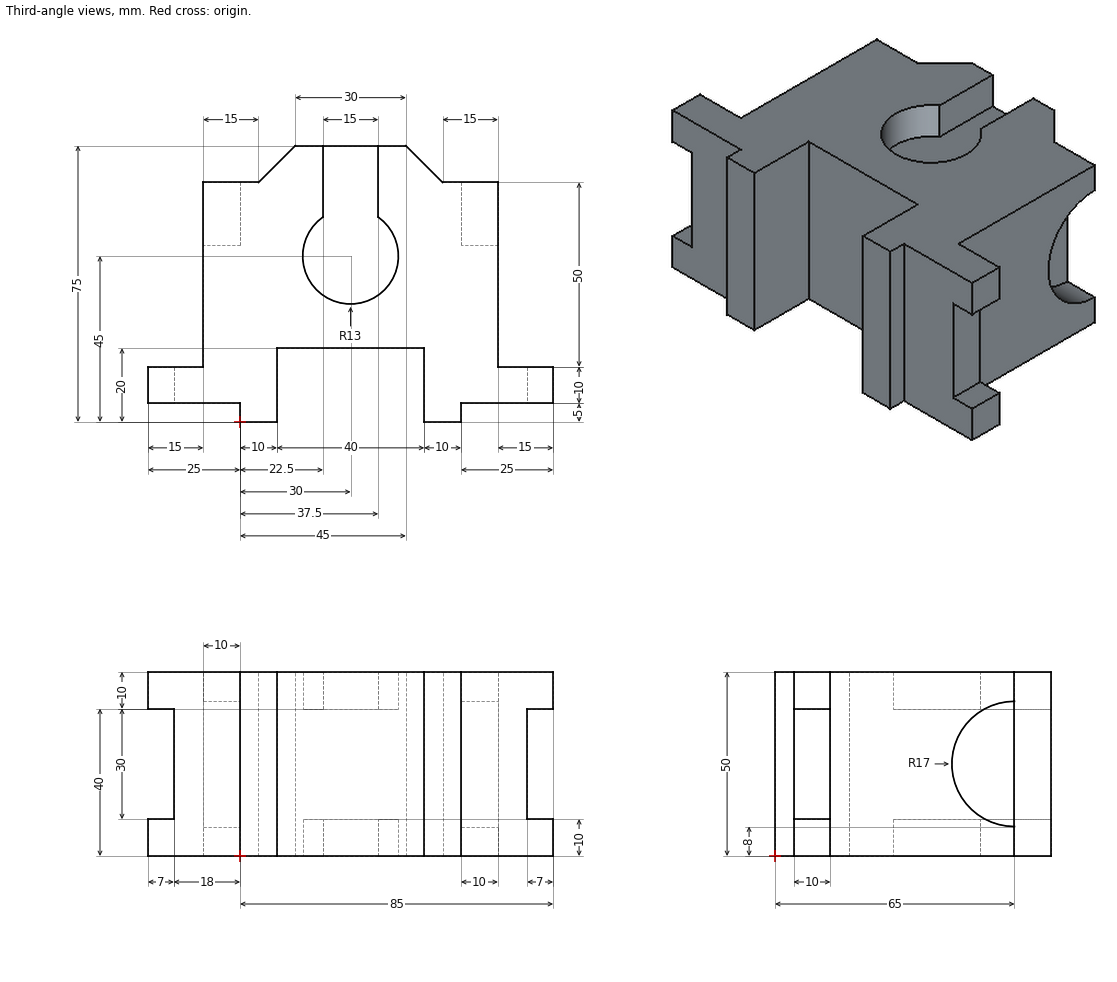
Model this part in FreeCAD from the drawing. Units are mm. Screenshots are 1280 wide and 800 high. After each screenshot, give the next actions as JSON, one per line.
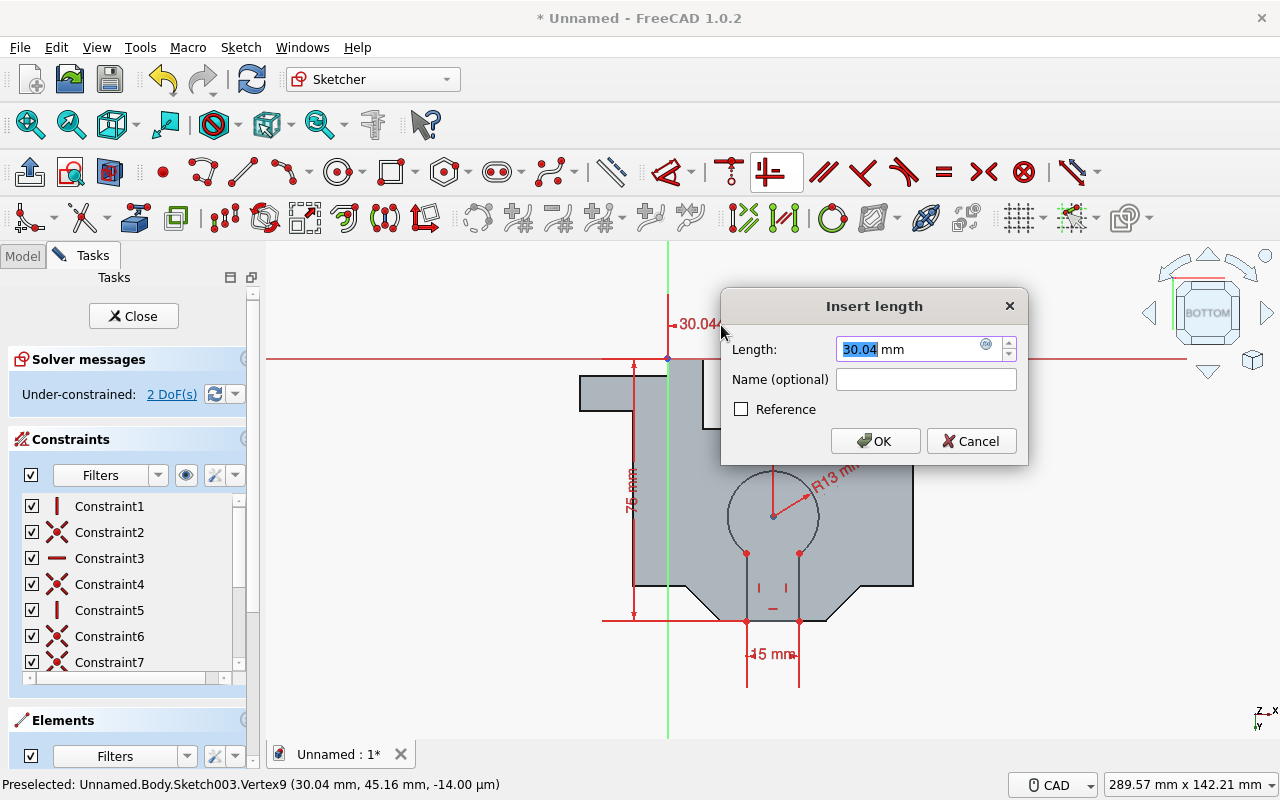
{"action": "type", "text": "30"}
{"action": "key", "text": "Return"}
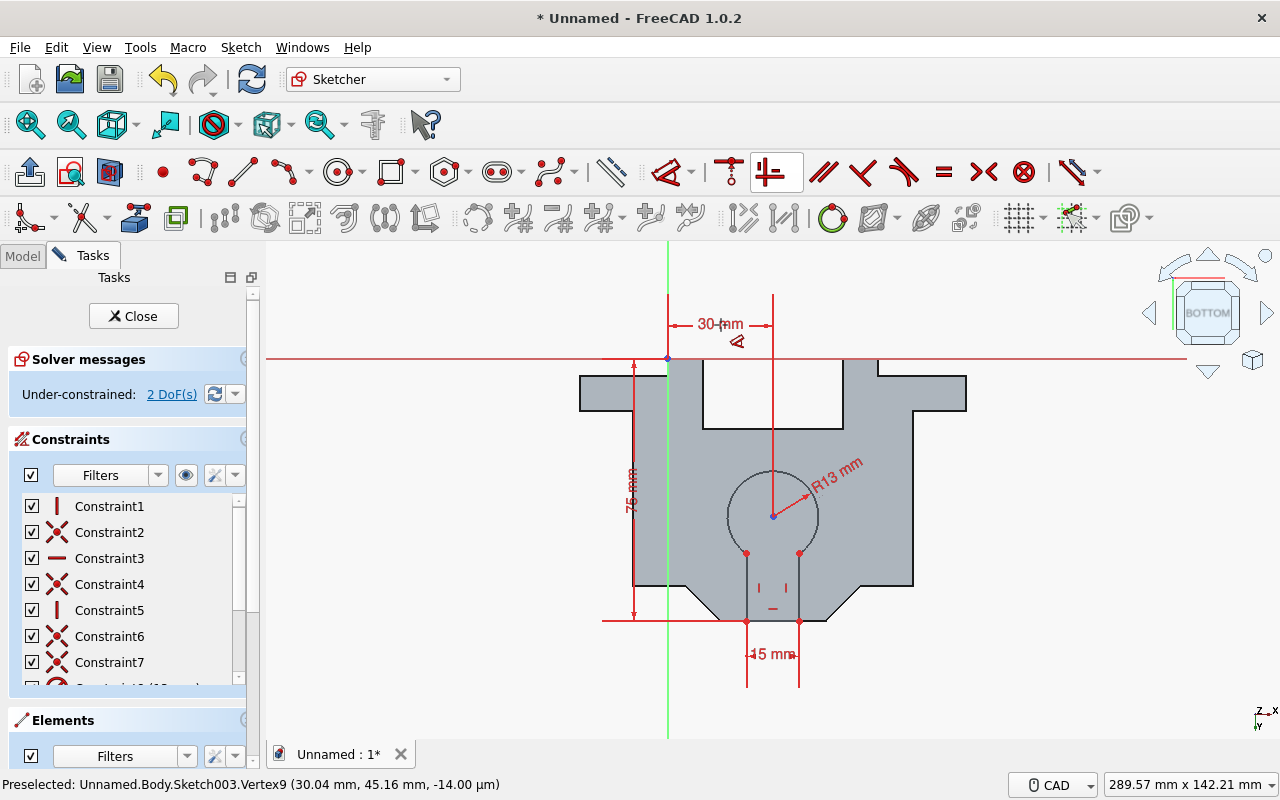
{"action": "left_click", "coordinate": [773, 517]}
{"action": "left_click", "coordinate": [634, 438]}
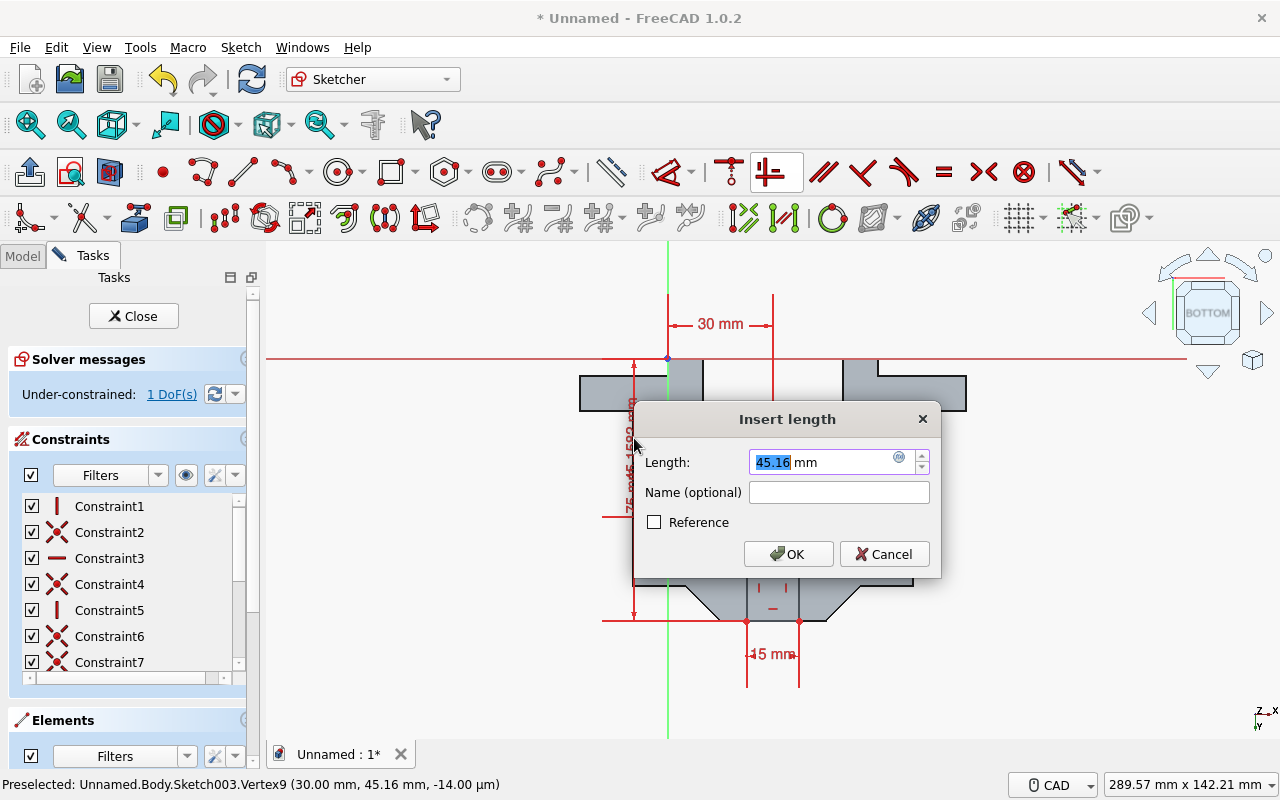
{"action": "type", "text": "45"}
{"action": "key", "text": "Return"}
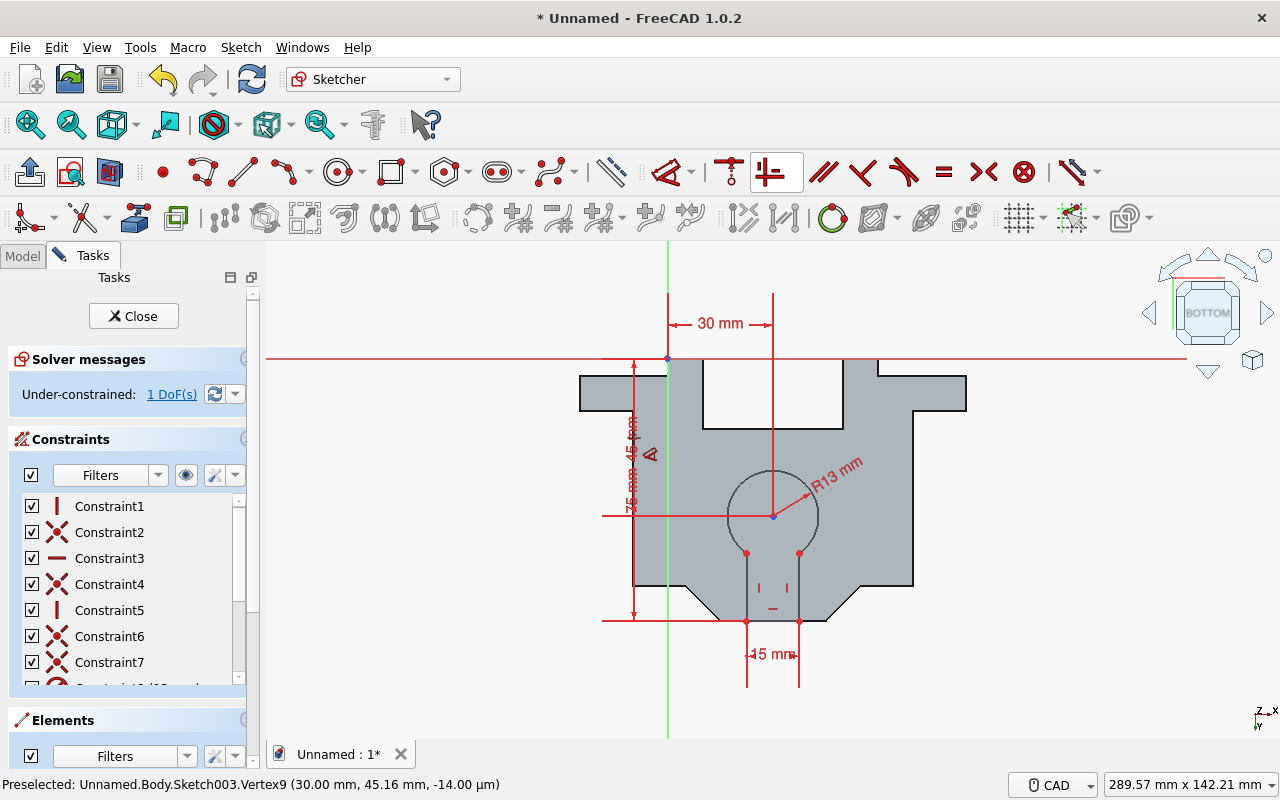
{"action": "left_click", "coordinate": [747, 554]}
{"action": "left_click", "coordinate": [707, 588]}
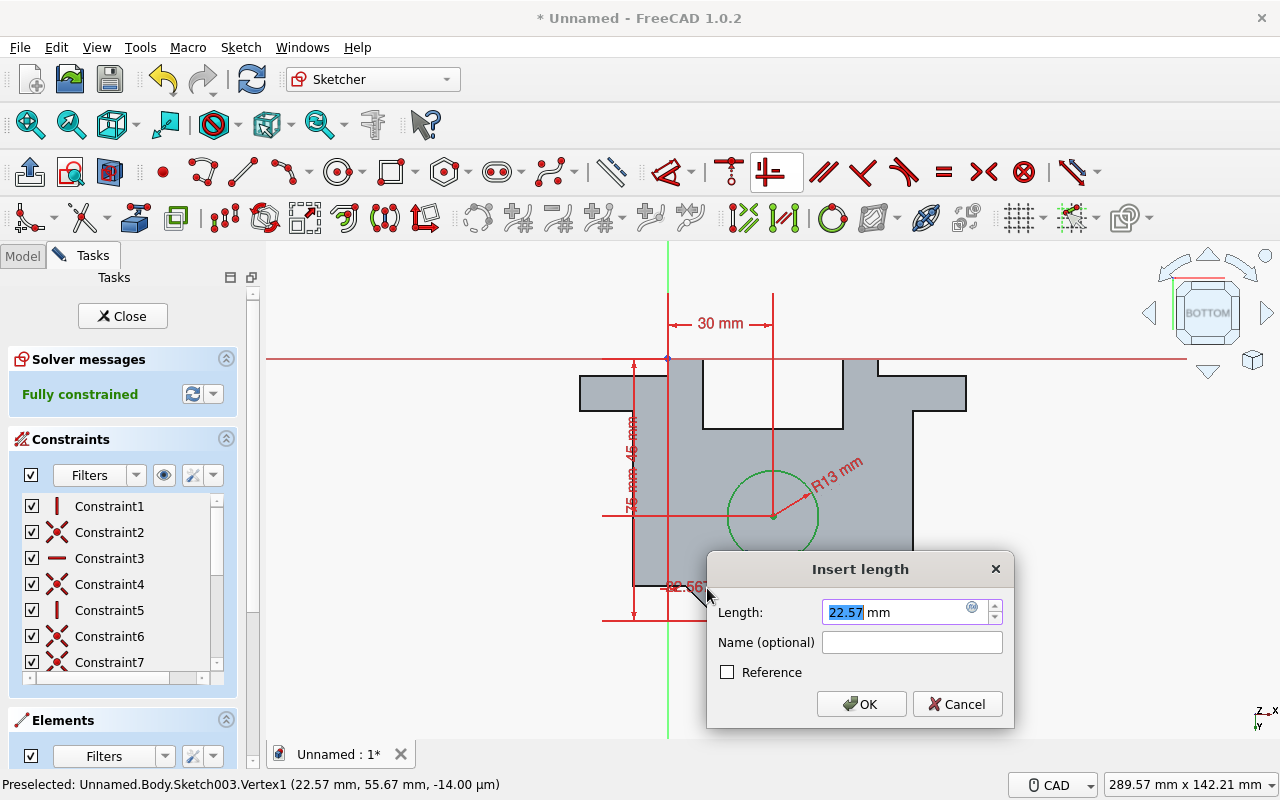
{"action": "type", "text": "22.5"}
{"action": "key", "text": "Return"}
{"action": "key", "text": "Escape"}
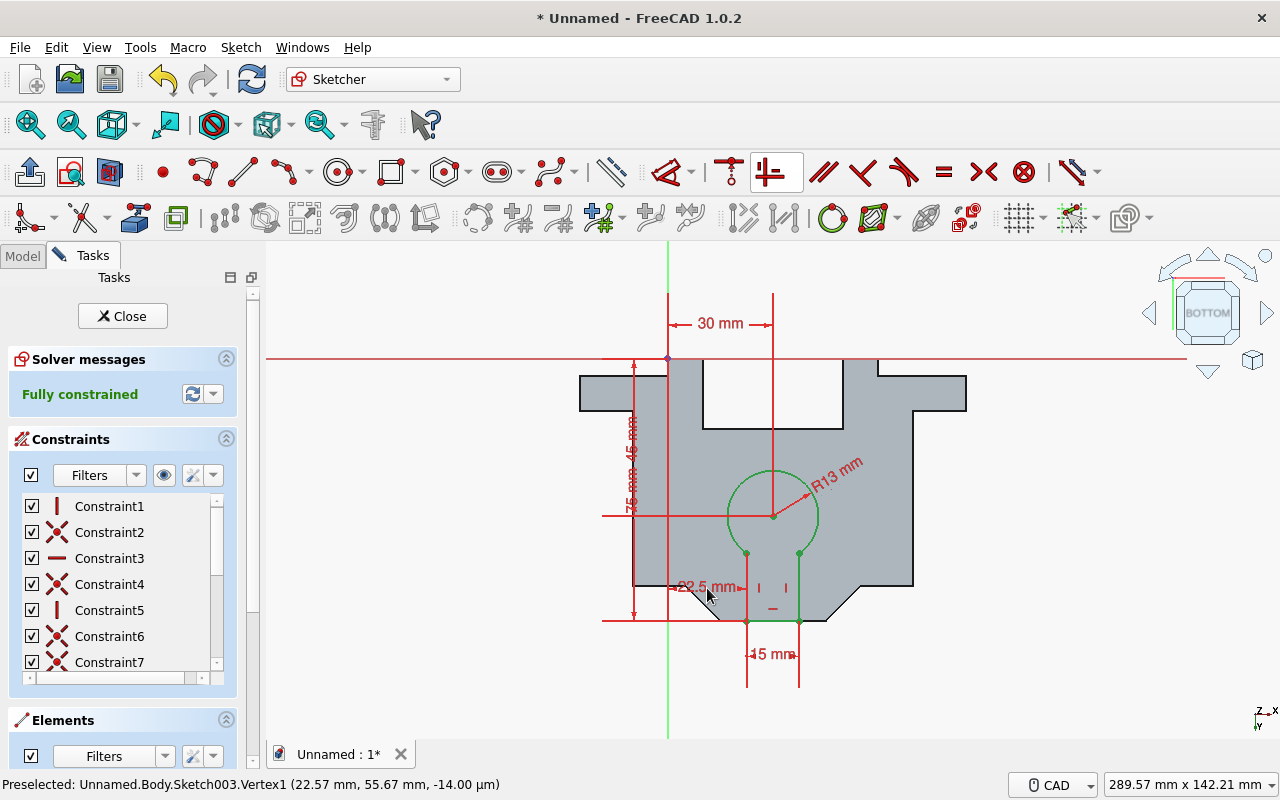
{"action": "left_click", "coordinate": [123, 316]}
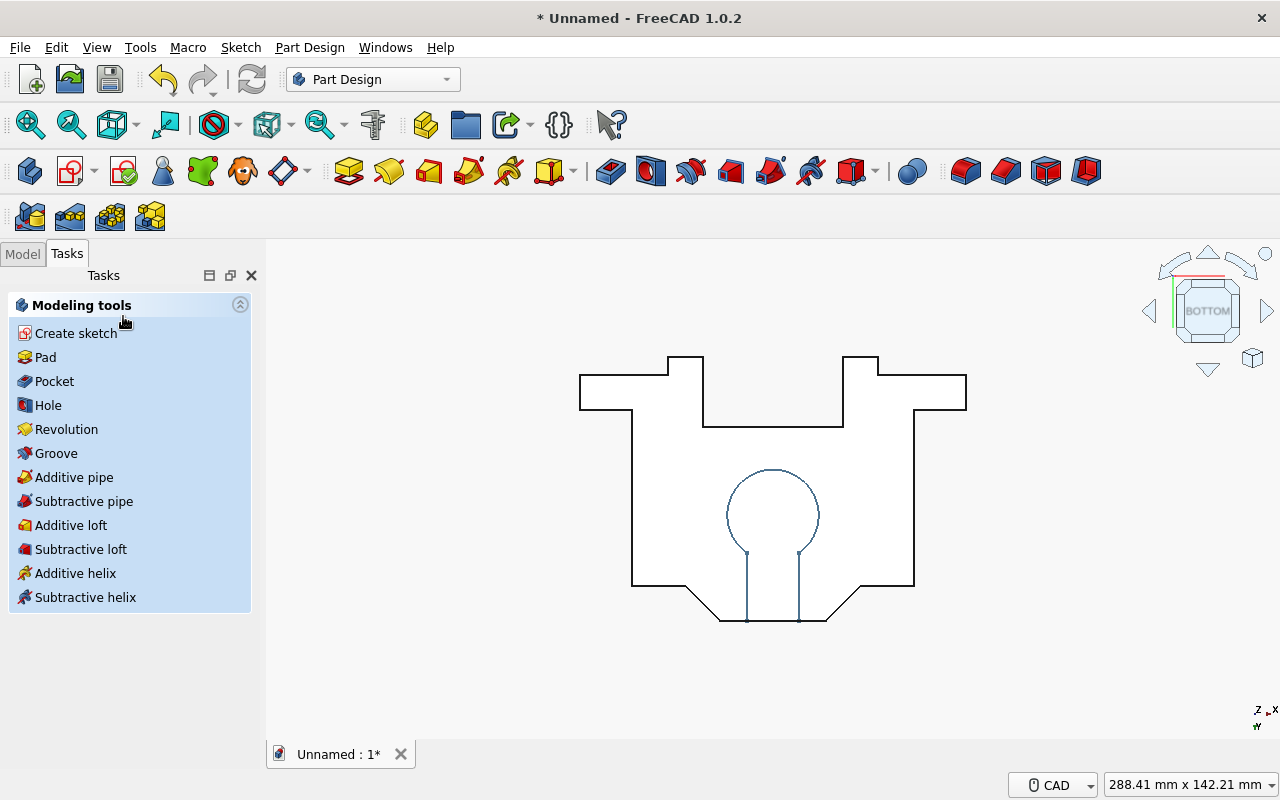
{"action": "left_click", "coordinate": [612, 172]}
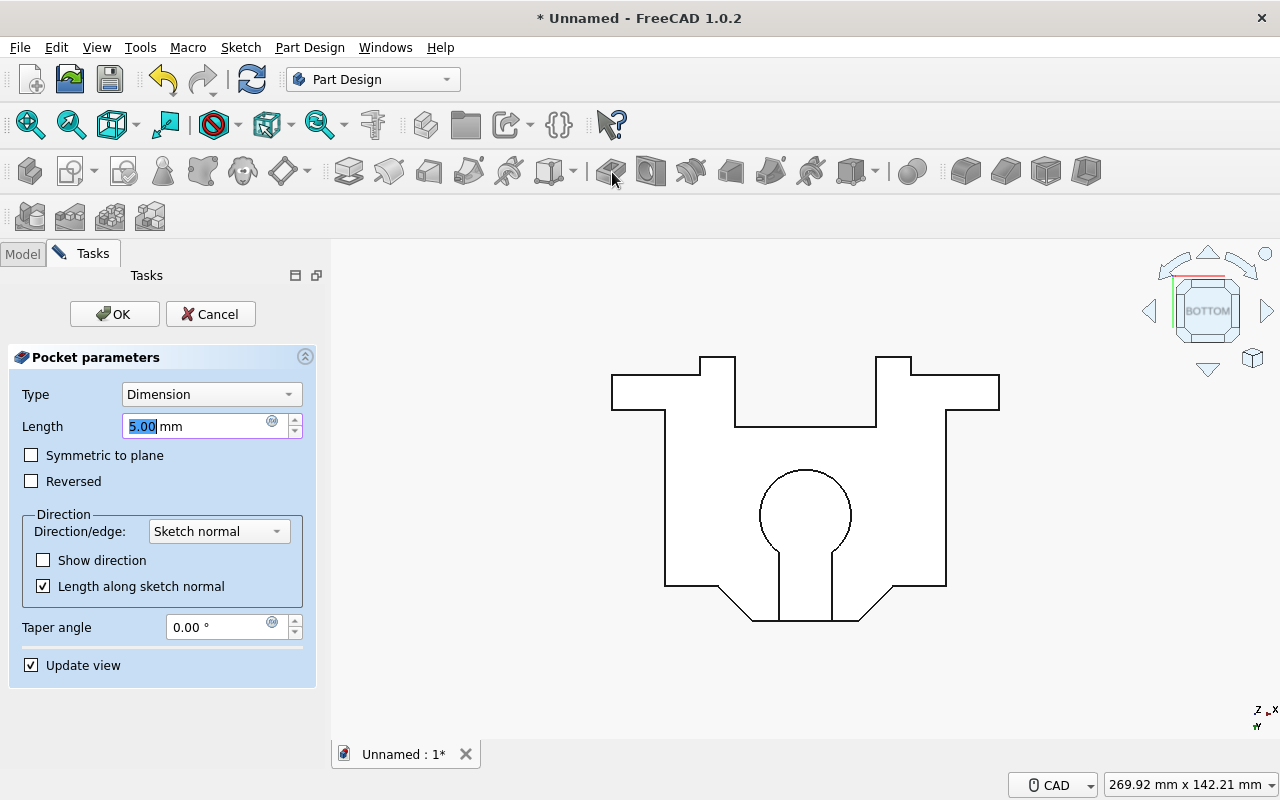
{"action": "type", "text": "10"}
{"action": "key", "text": "Tab"}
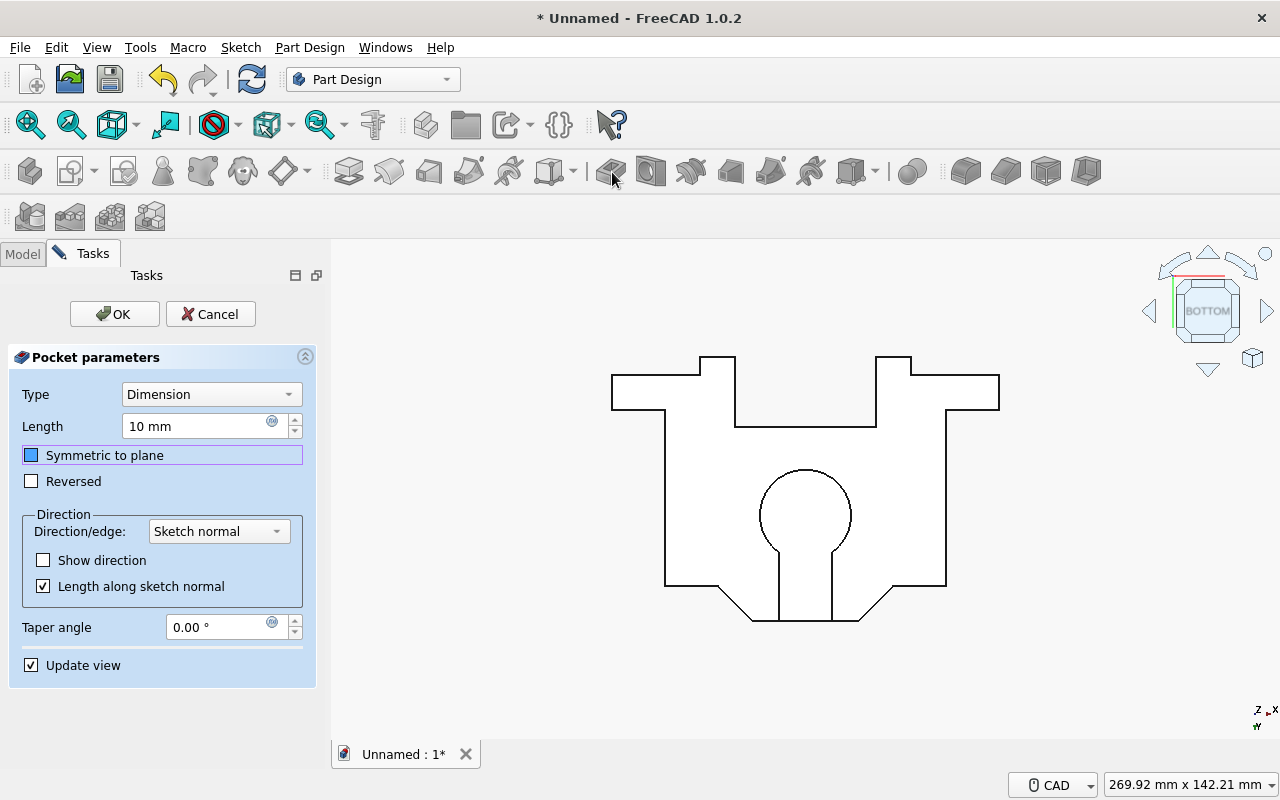
{"action": "left_click", "coordinate": [115, 314]}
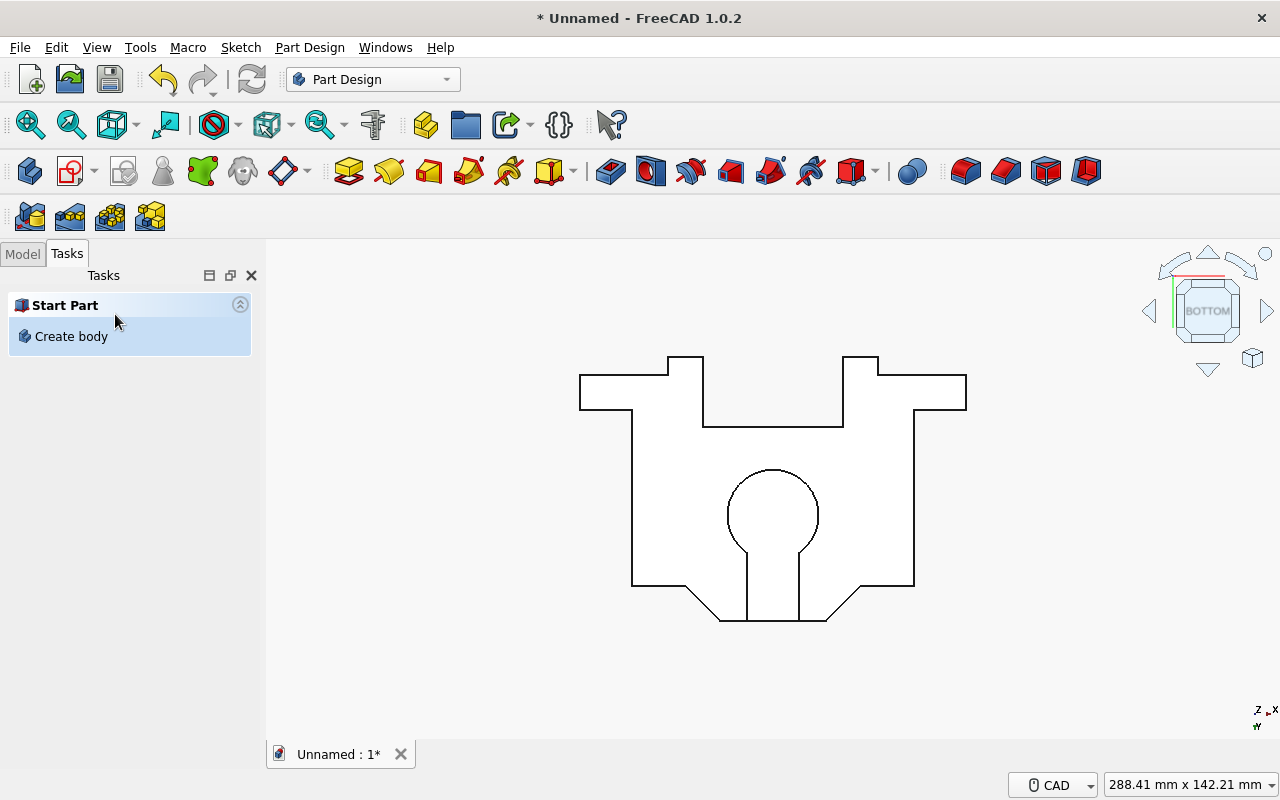
{"action": "left_click", "coordinate": [23, 253]}